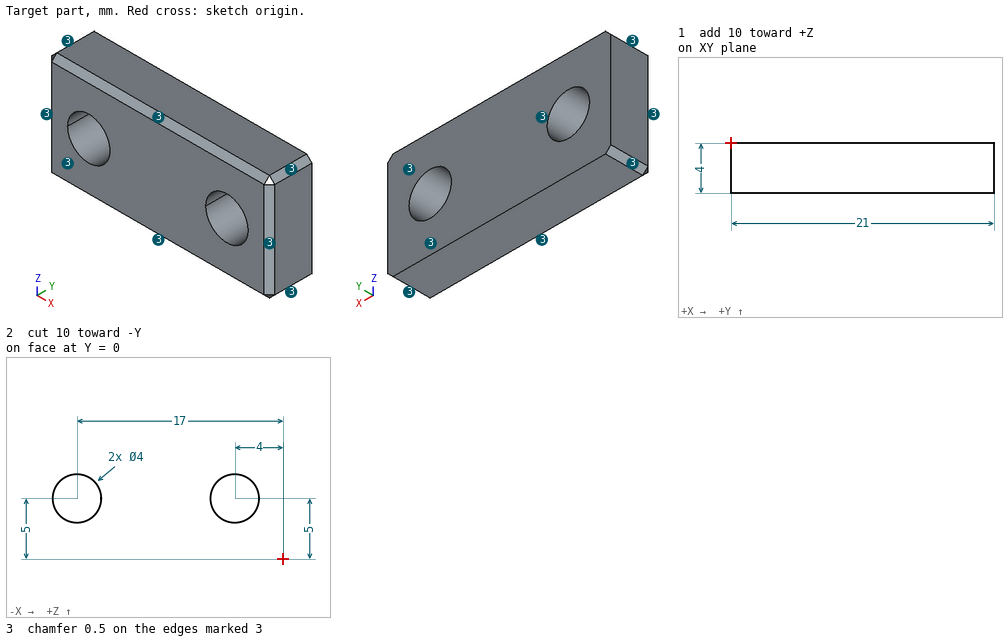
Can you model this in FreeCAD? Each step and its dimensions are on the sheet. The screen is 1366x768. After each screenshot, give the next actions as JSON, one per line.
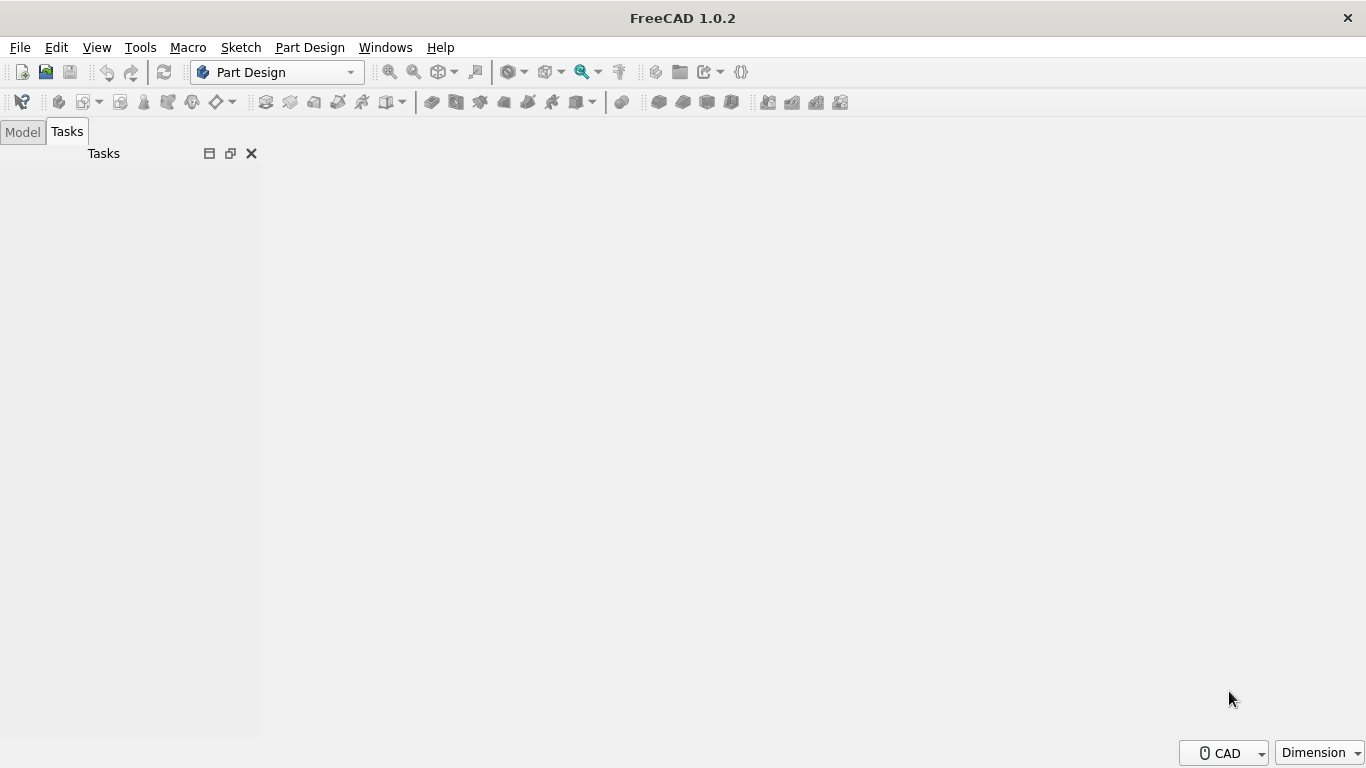
{"action": "left_click", "coordinate": [22, 72]}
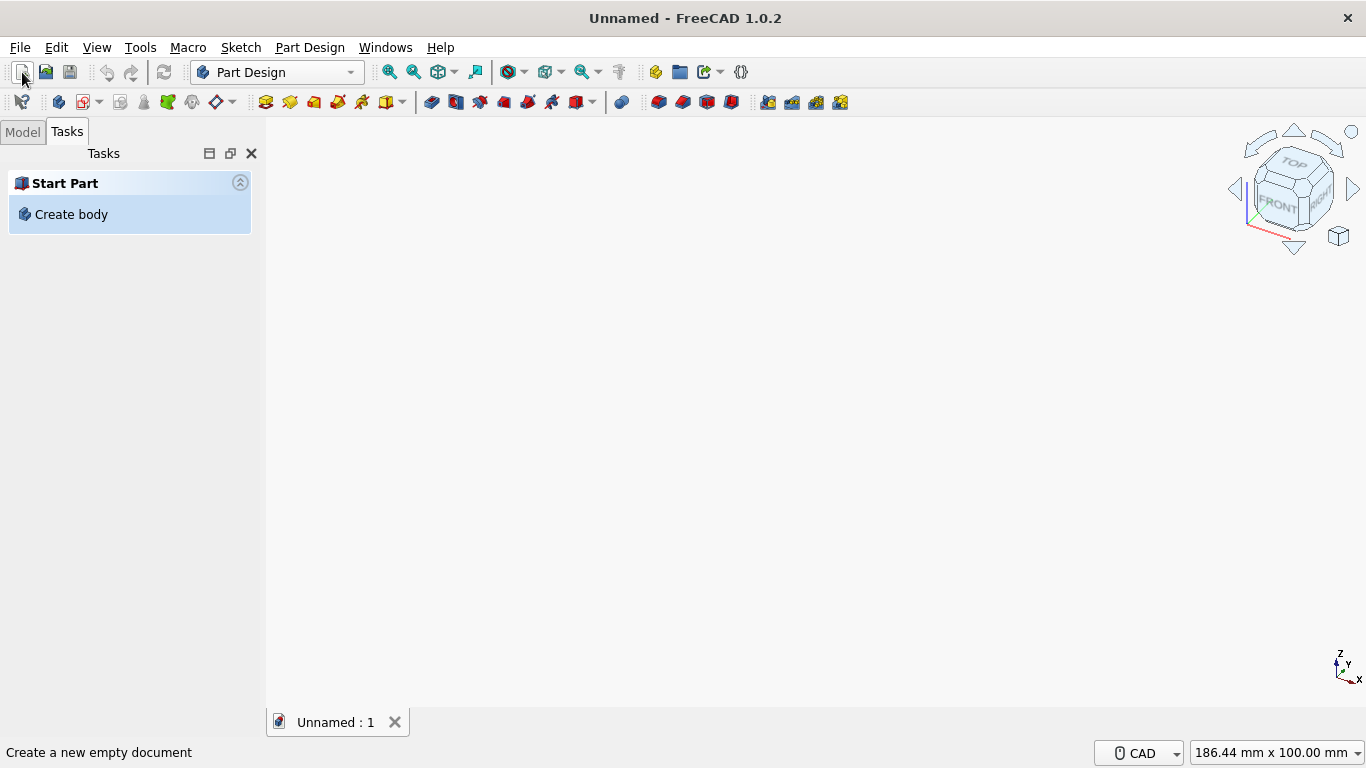
{"action": "left_click", "coordinate": [84, 102]}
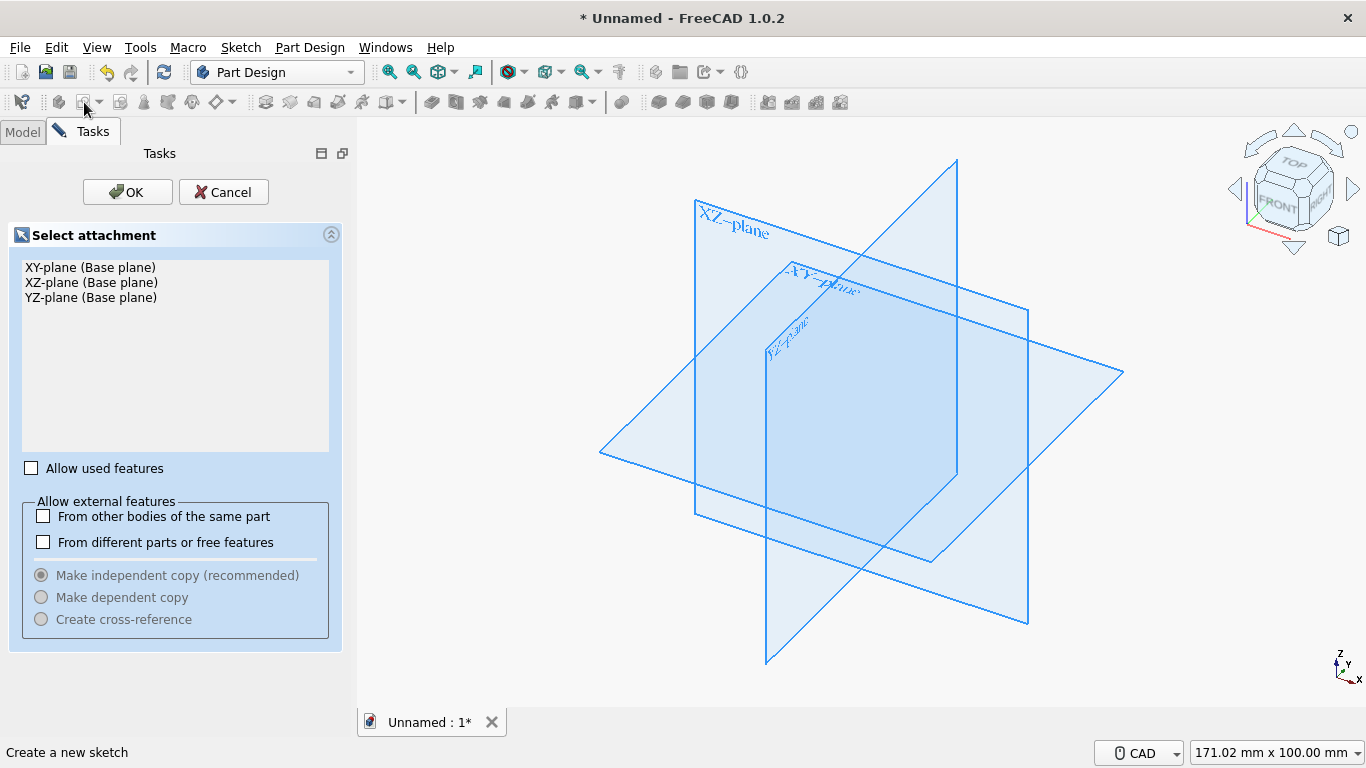
{"action": "left_click", "coordinate": [82, 268]}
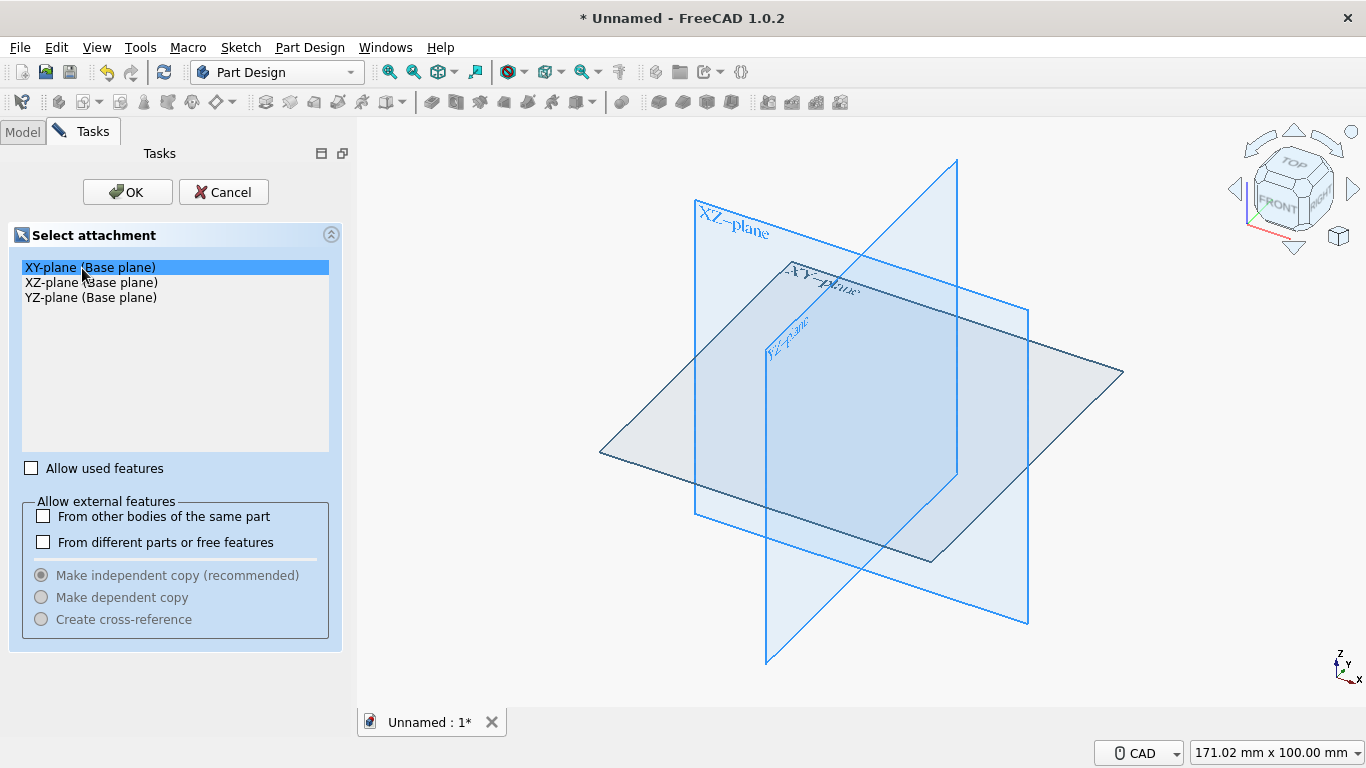
{"action": "left_click", "coordinate": [128, 192]}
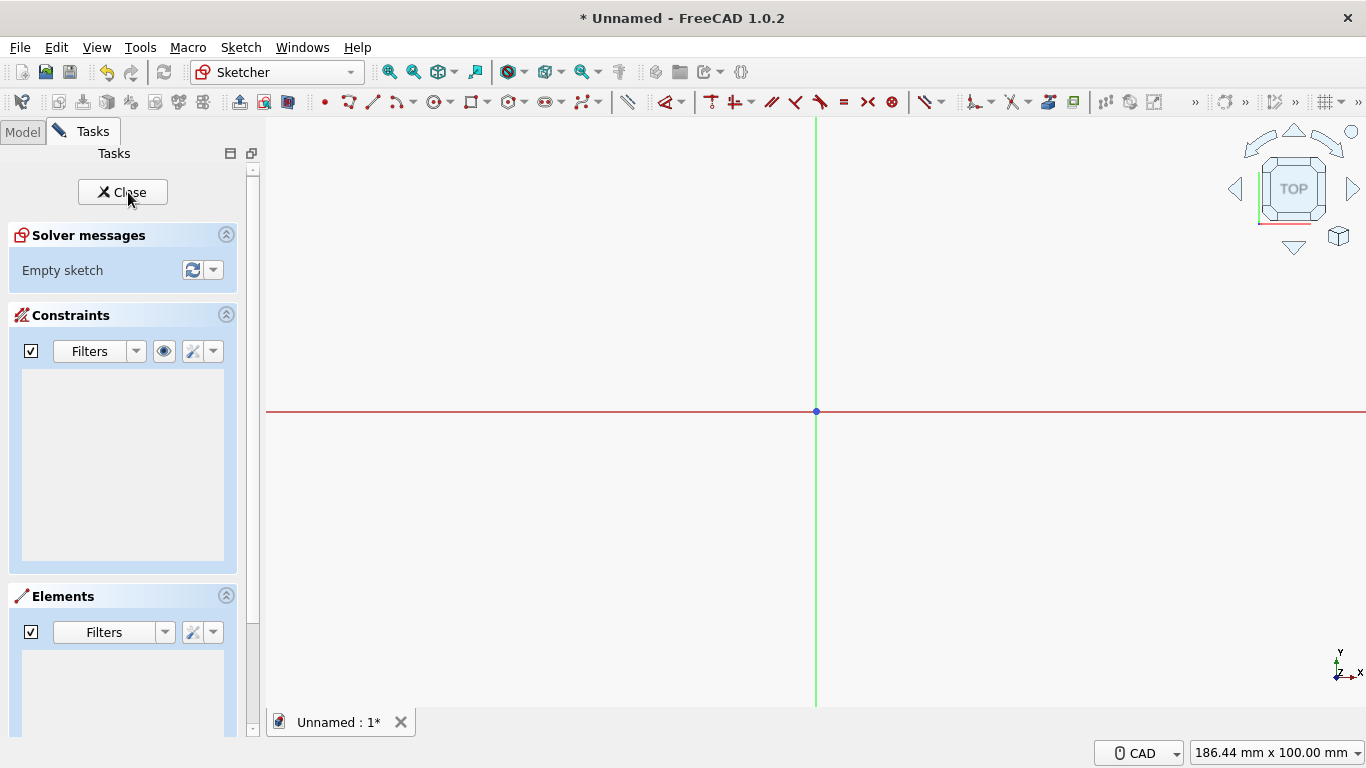
{"action": "scroll", "coordinate": [911, 427], "scroll_direction": "up", "scroll_amount": 8}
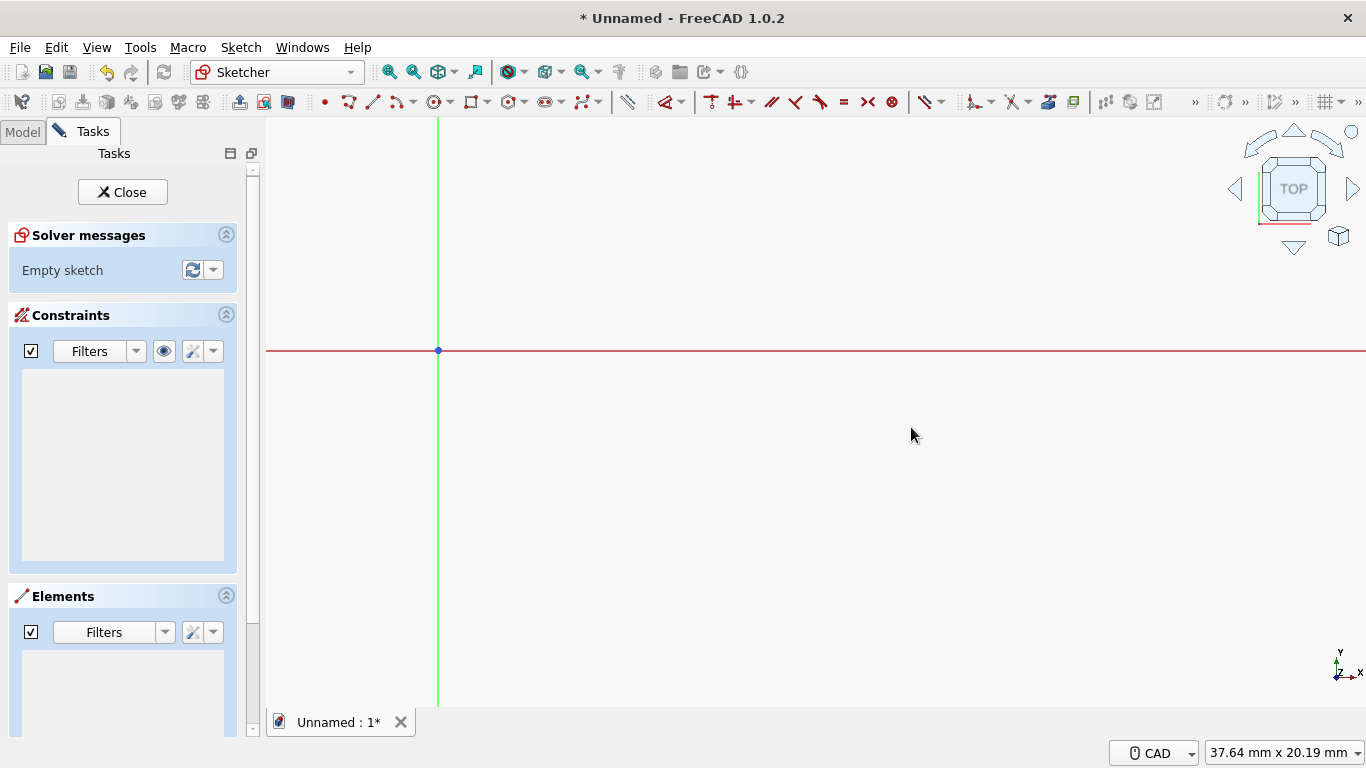
{"action": "left_click", "coordinate": [472, 102]}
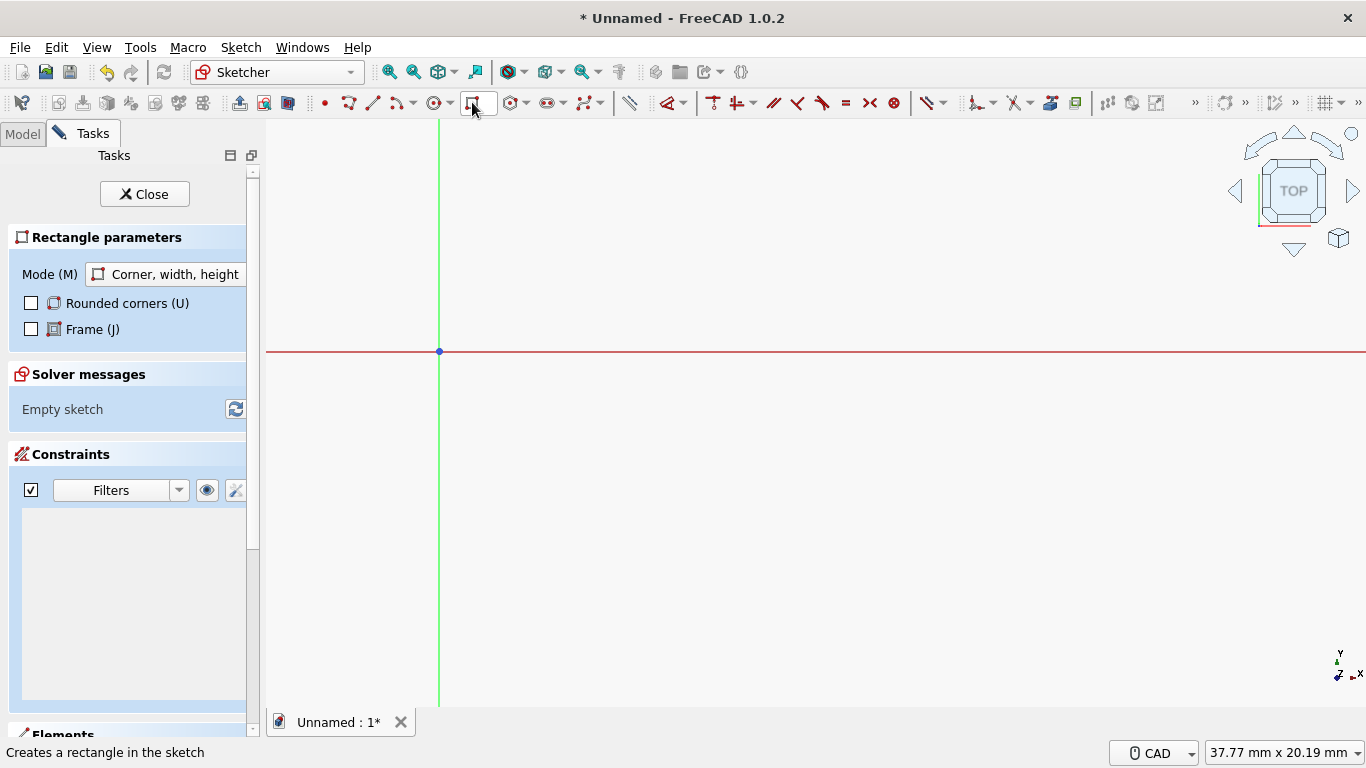
{"action": "left_click", "coordinate": [439, 352]}
{"action": "left_click", "coordinate": [1051, 468]}
{"action": "key", "text": "Escape"}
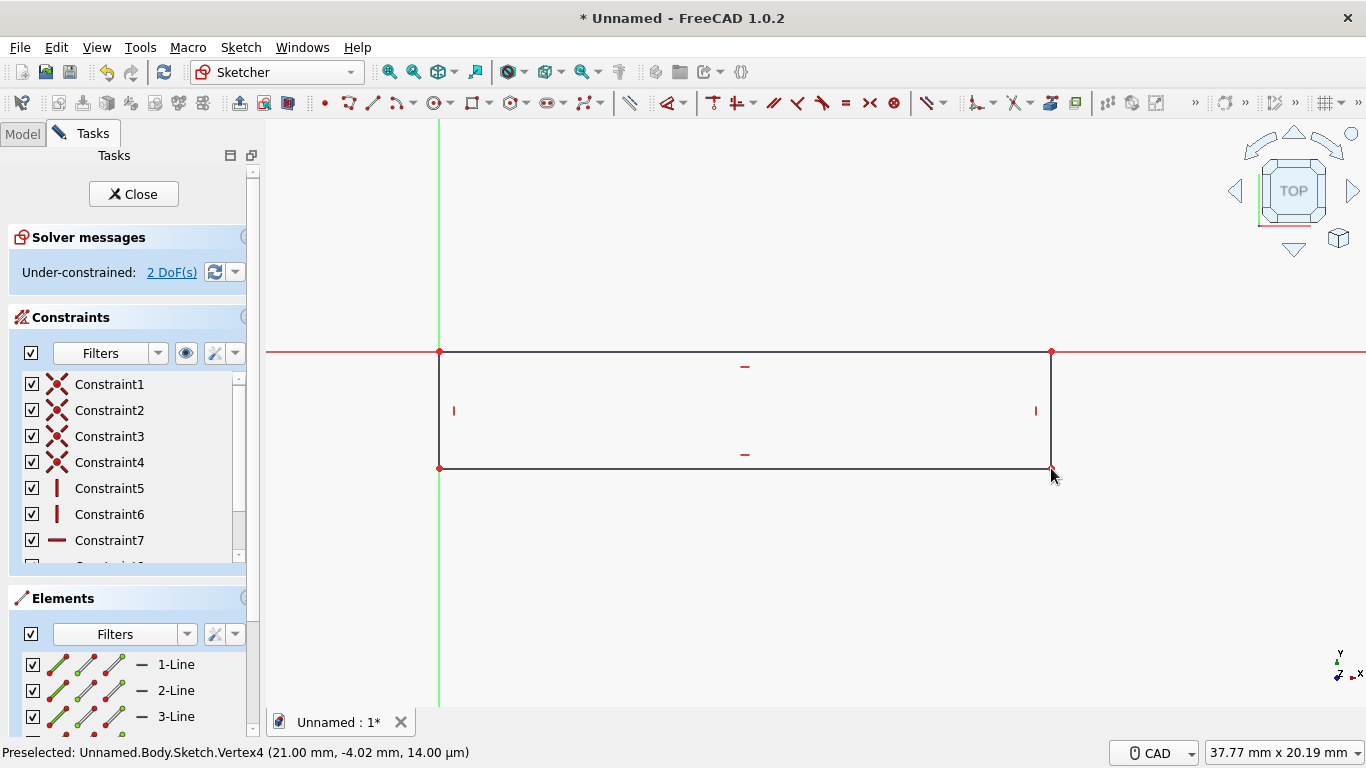
{"action": "left_click", "coordinate": [668, 104]}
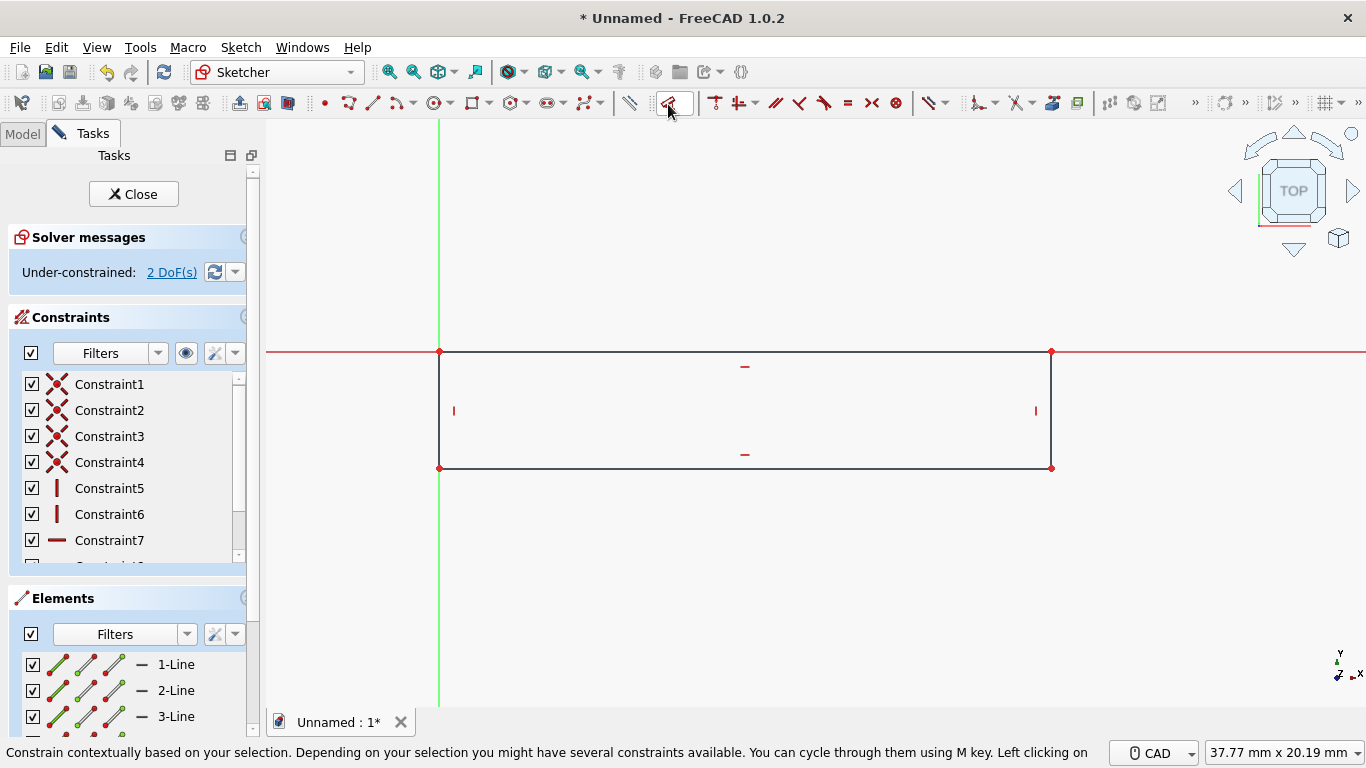
{"action": "left_click", "coordinate": [439, 387]}
{"action": "left_click", "coordinate": [405, 410]}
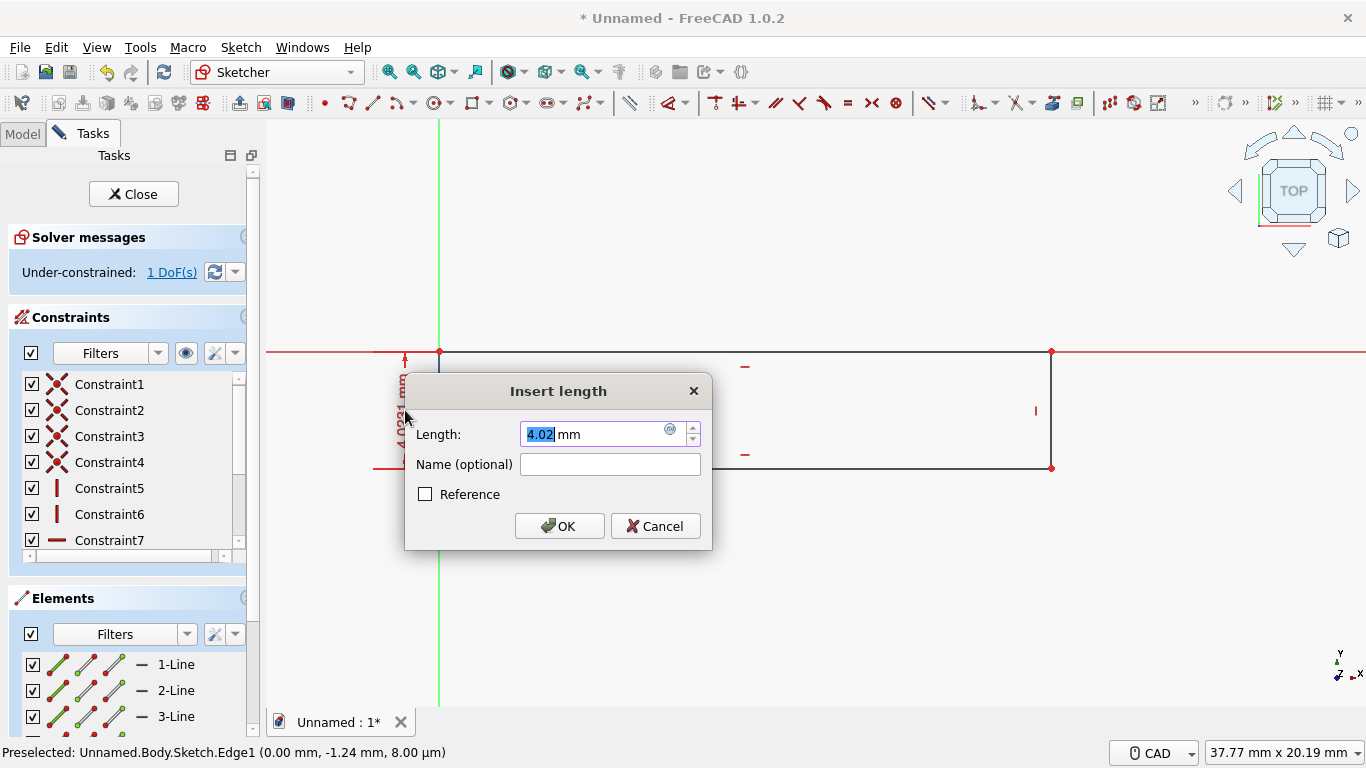
{"action": "type", "text": "4"}
{"action": "key", "text": "Return"}